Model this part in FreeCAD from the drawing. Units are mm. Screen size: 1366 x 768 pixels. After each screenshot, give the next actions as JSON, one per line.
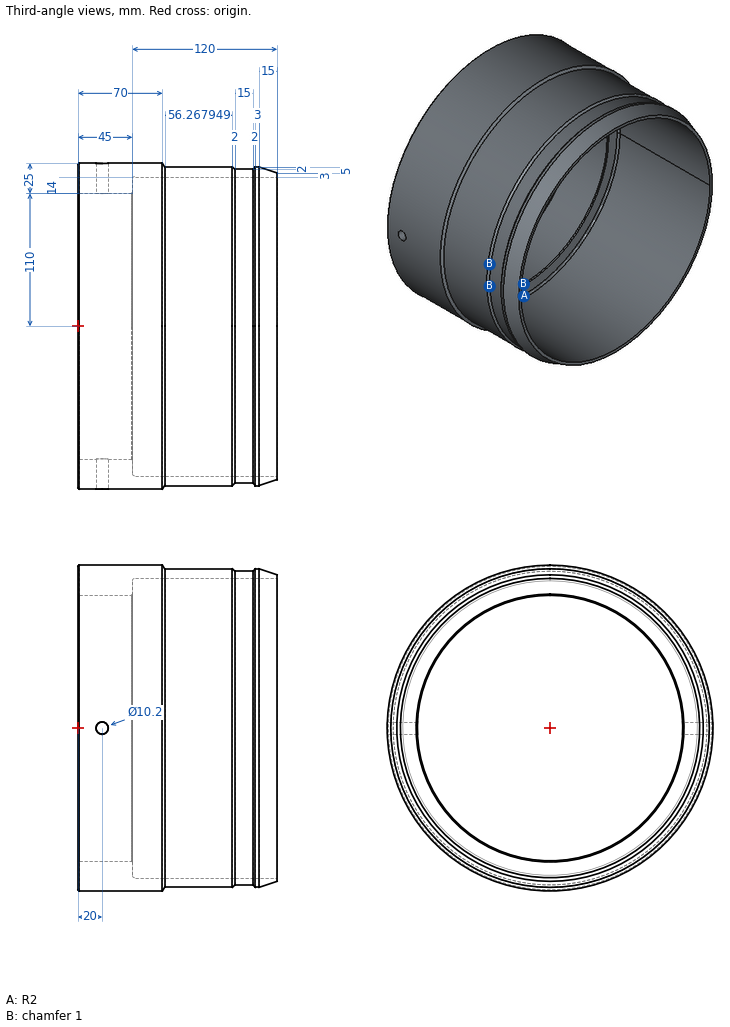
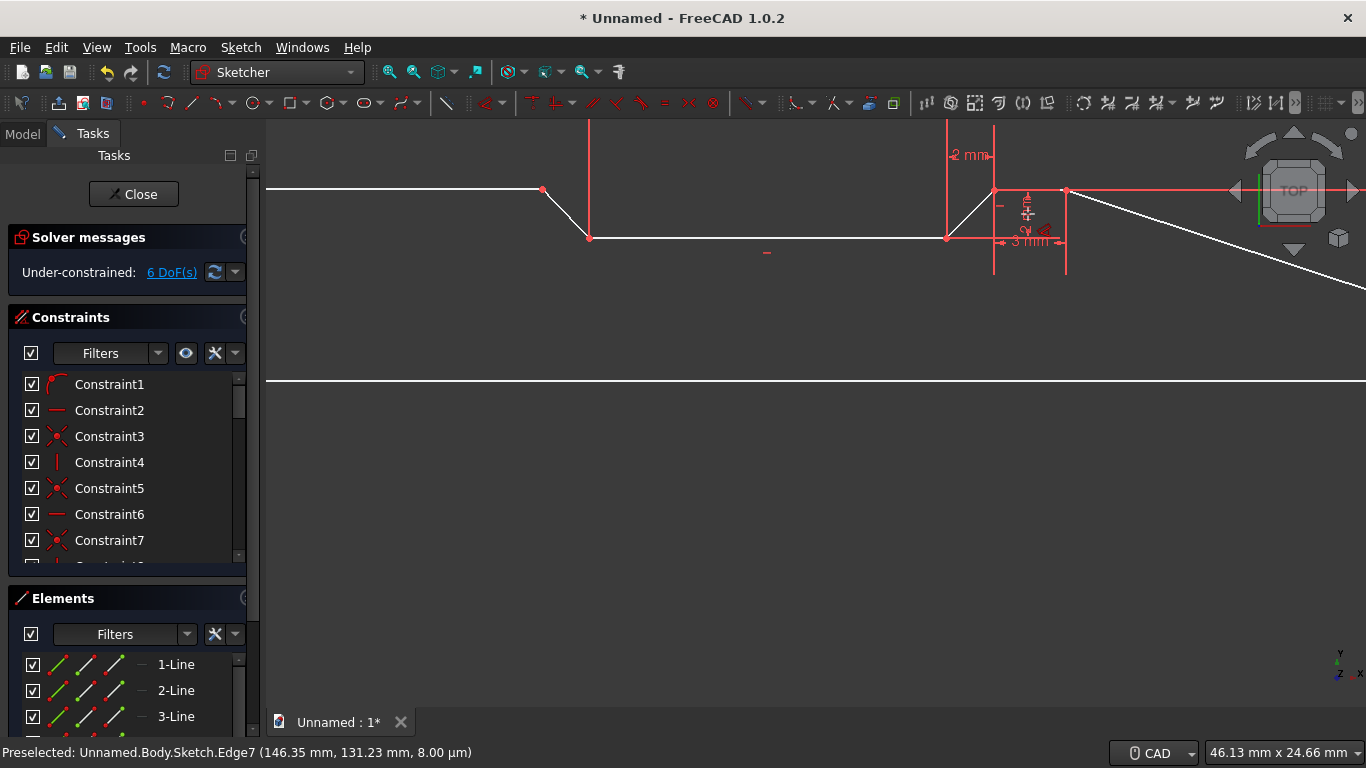
{"action": "left_click", "coordinate": [575, 223]}
{"action": "left_click", "coordinate": [566, 155]}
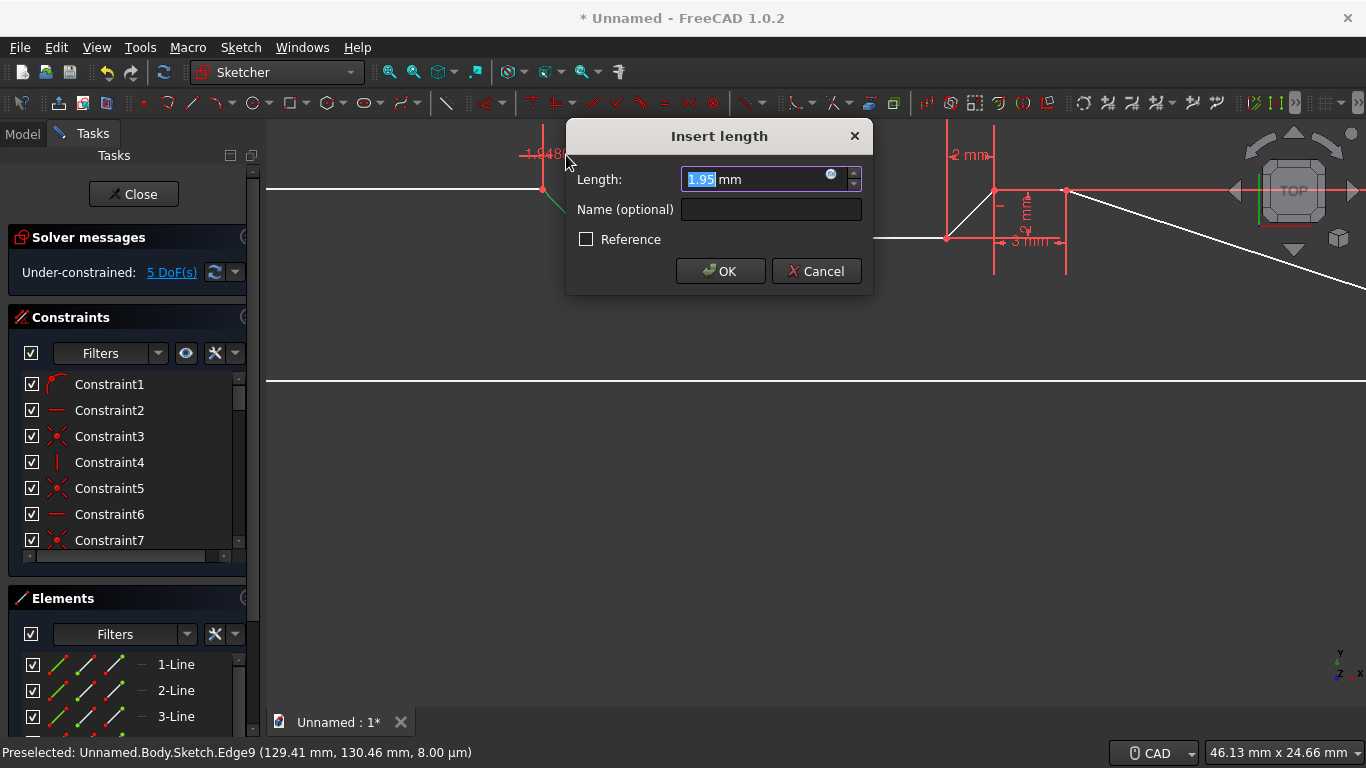
{"action": "type", "text": "2"}
{"action": "key", "text": "Return"}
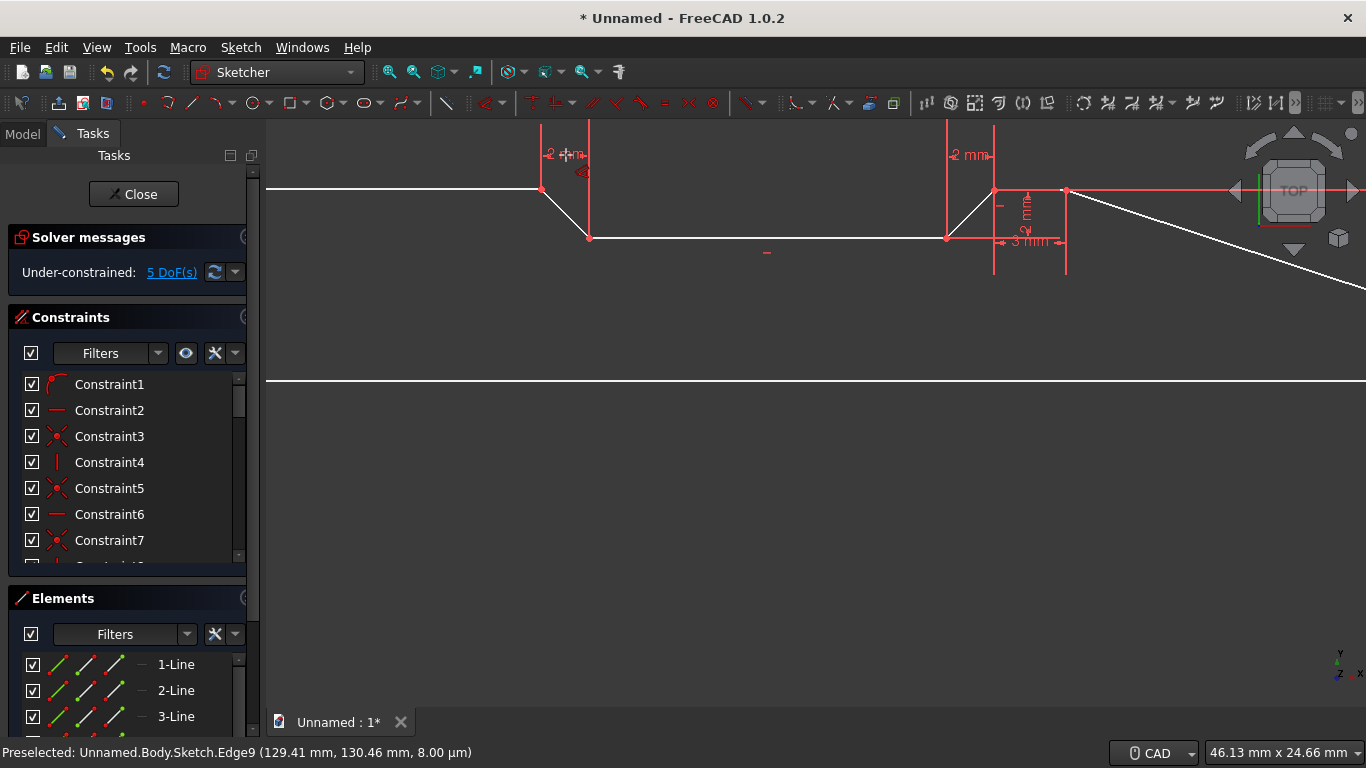
{"action": "left_click", "coordinate": [575, 223]}
{"action": "left_click", "coordinate": [623, 214]}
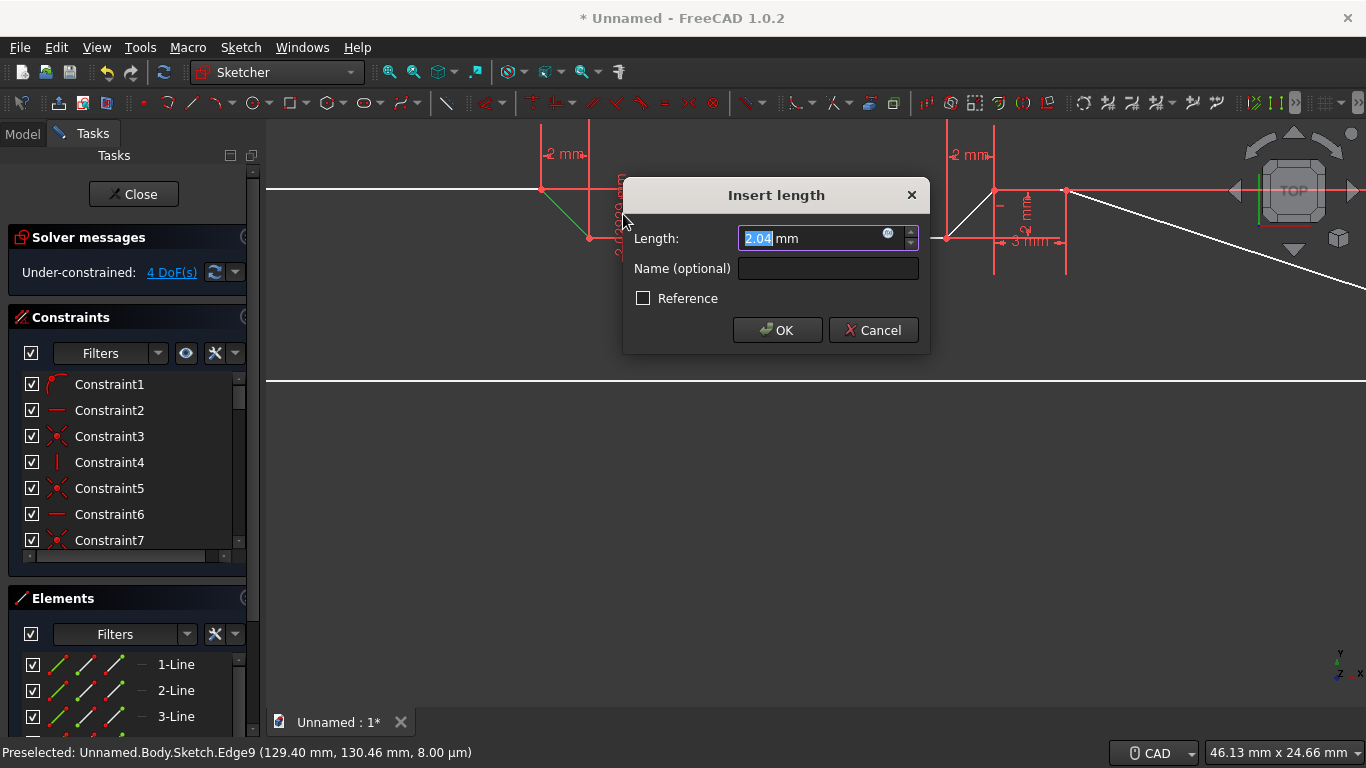
{"action": "type", "text": "2"}
{"action": "key", "text": "Return"}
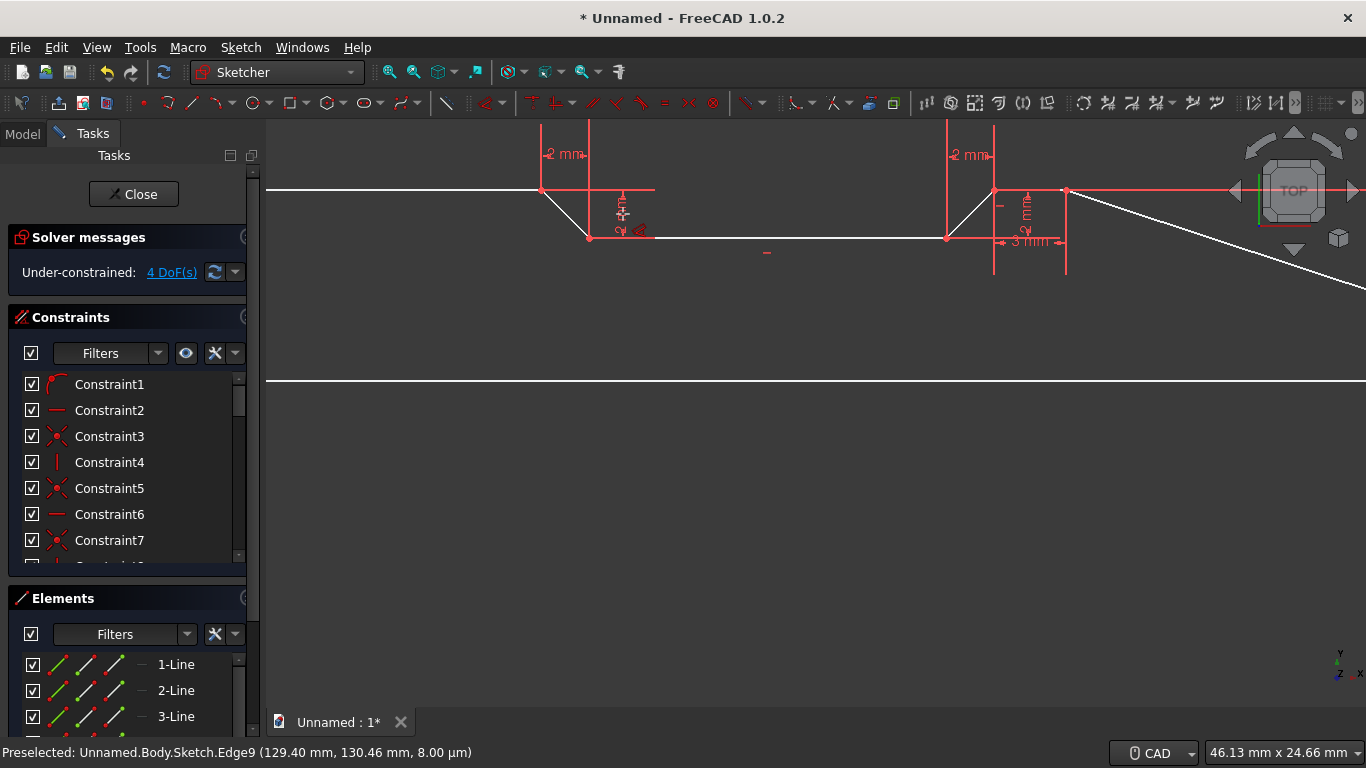
{"action": "scroll", "coordinate": [908, 250], "scroll_direction": "down", "scroll_amount": 11}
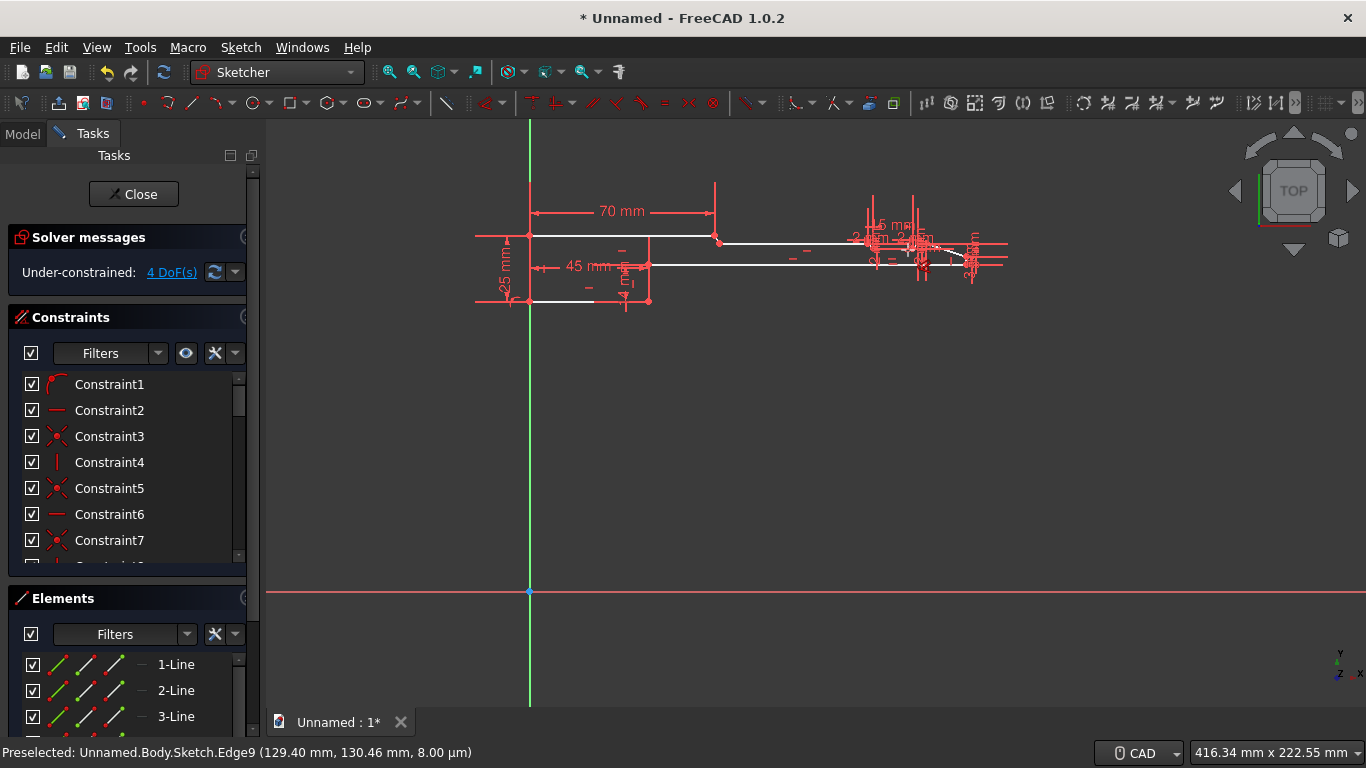
{"action": "left_click", "coordinate": [871, 265]}
{"action": "left_click", "coordinate": [807, 299]}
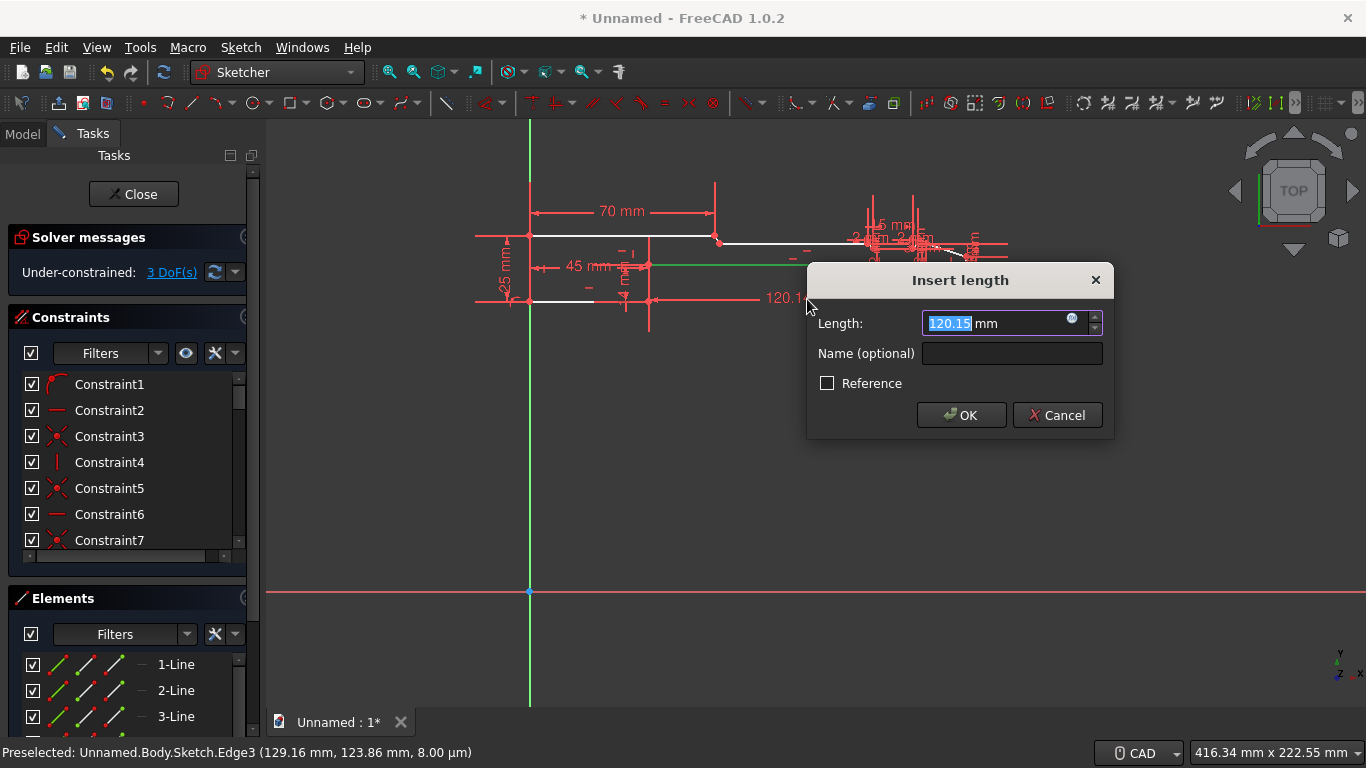
{"action": "type", "text": "120"}
{"action": "key", "text": "Return"}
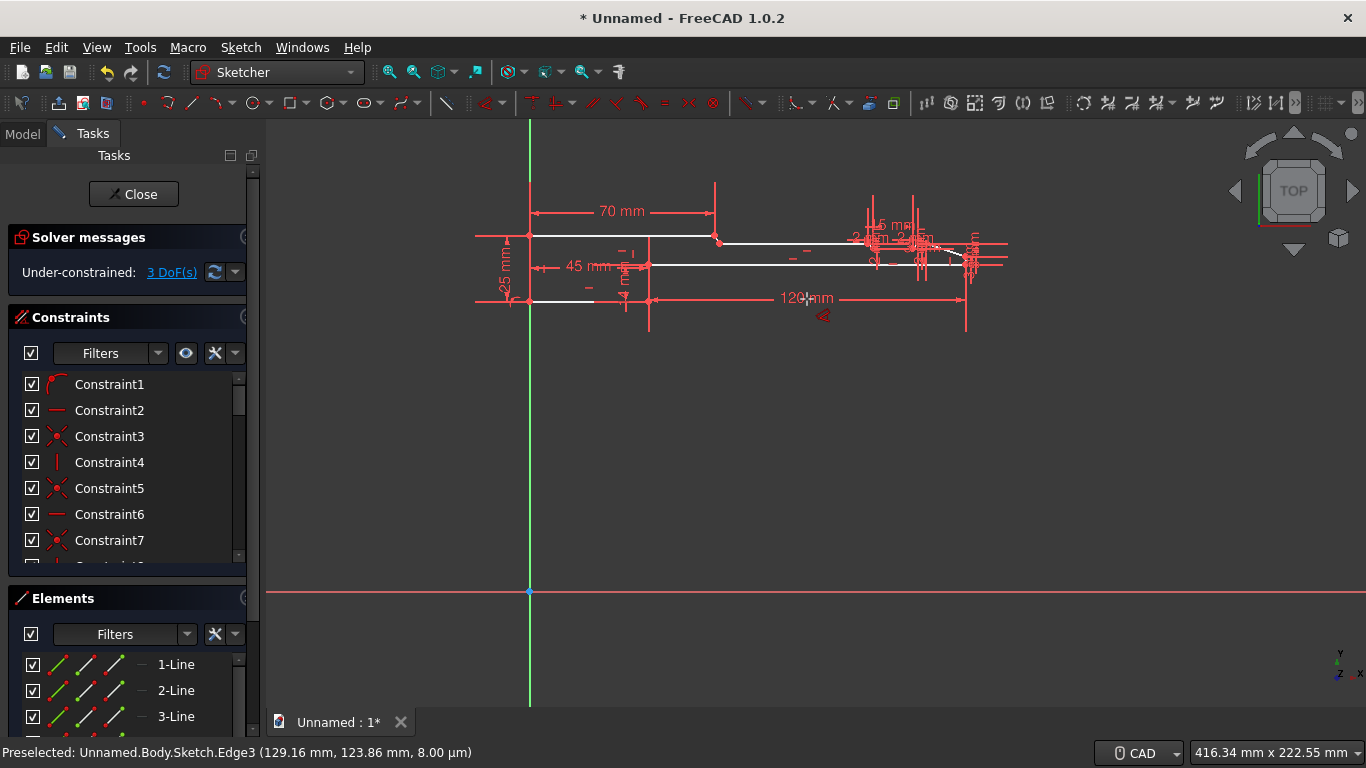
{"action": "left_click", "coordinate": [954, 253]}
{"action": "left_click", "coordinate": [946, 291]}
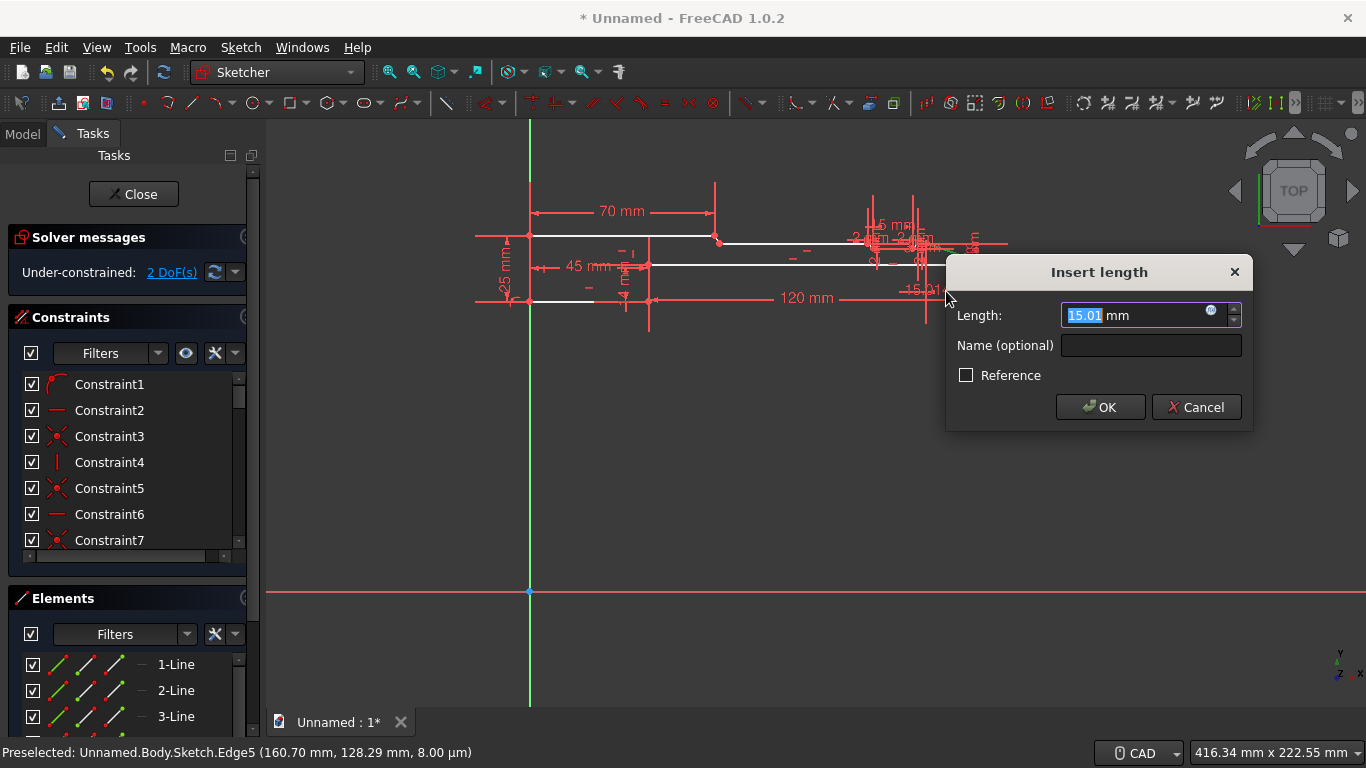
{"action": "type", "text": "15"}
{"action": "key", "text": "Return"}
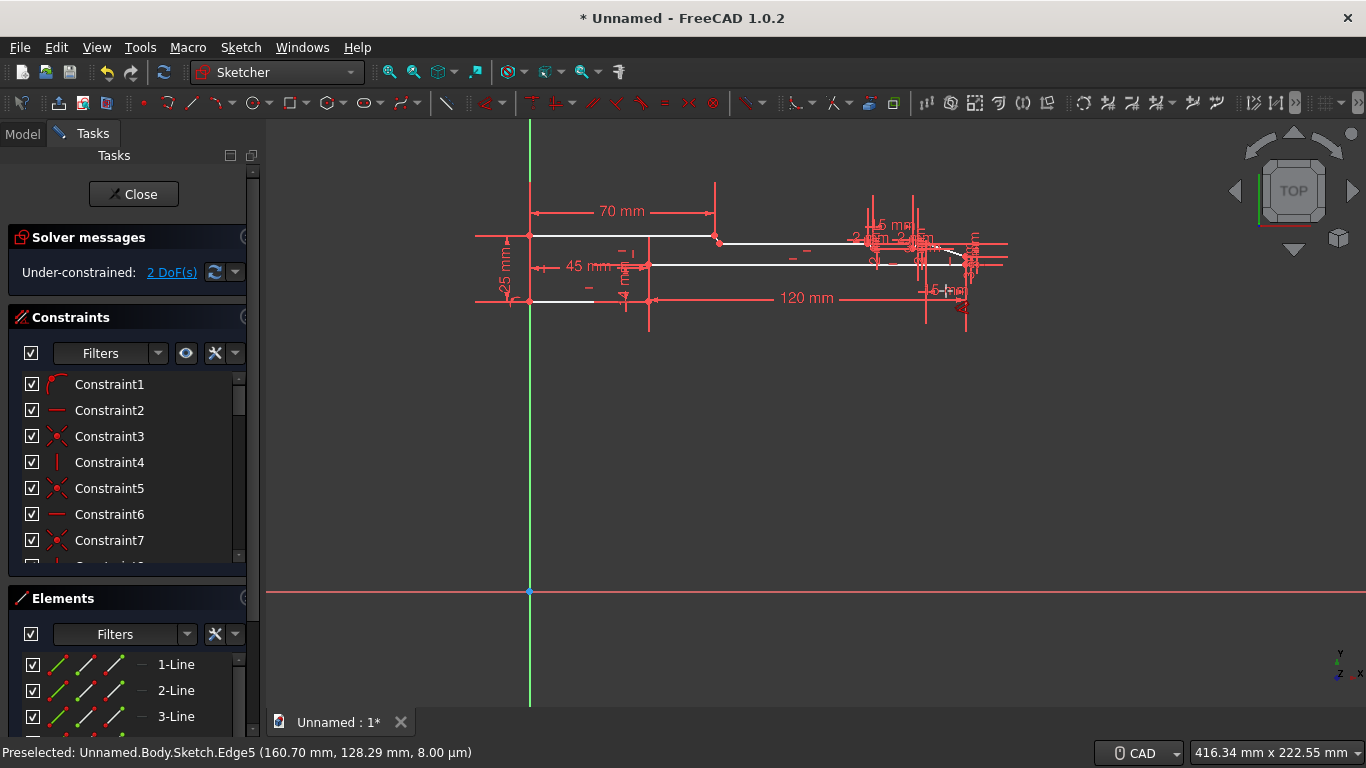
{"action": "left_click", "coordinate": [530, 302]}
{"action": "left_click", "coordinate": [496, 447]}